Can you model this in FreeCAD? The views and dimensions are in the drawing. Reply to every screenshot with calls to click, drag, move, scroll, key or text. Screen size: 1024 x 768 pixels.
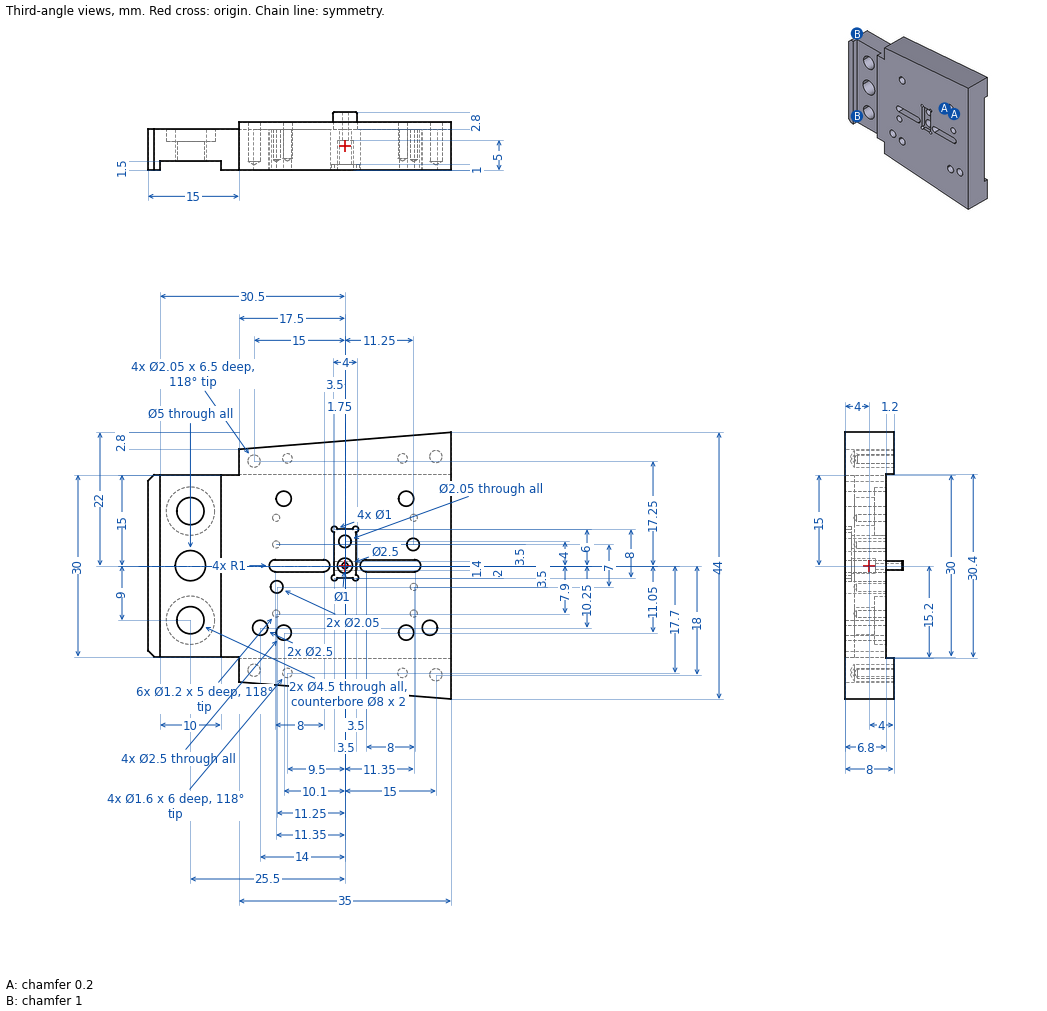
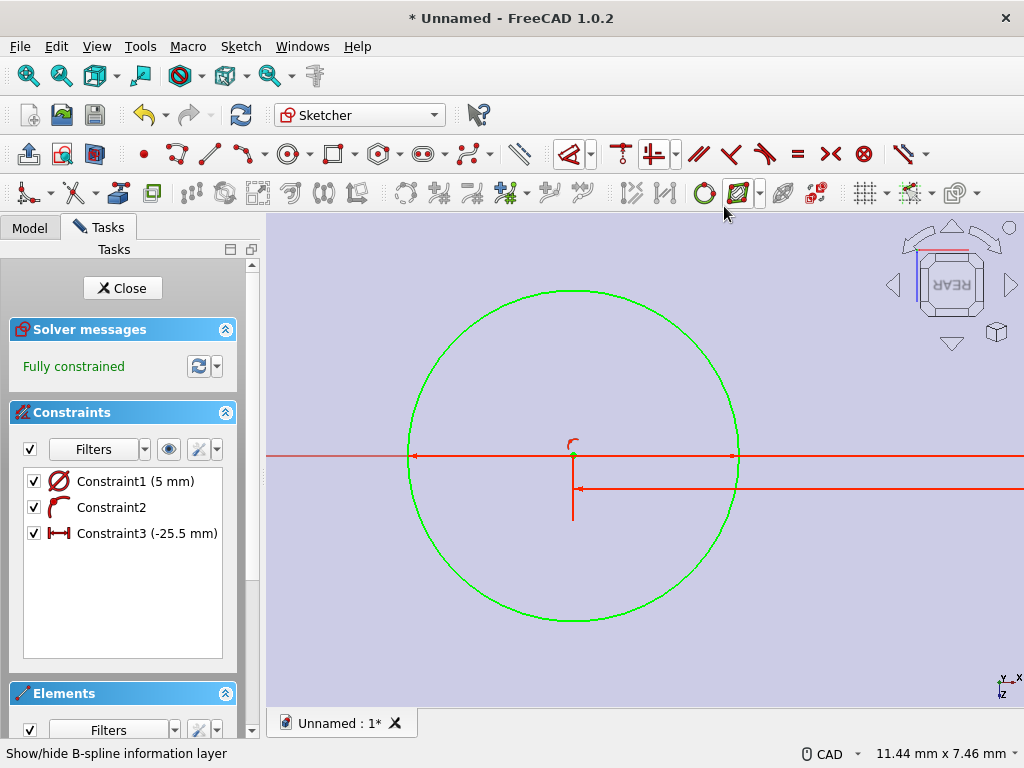
click(123, 288)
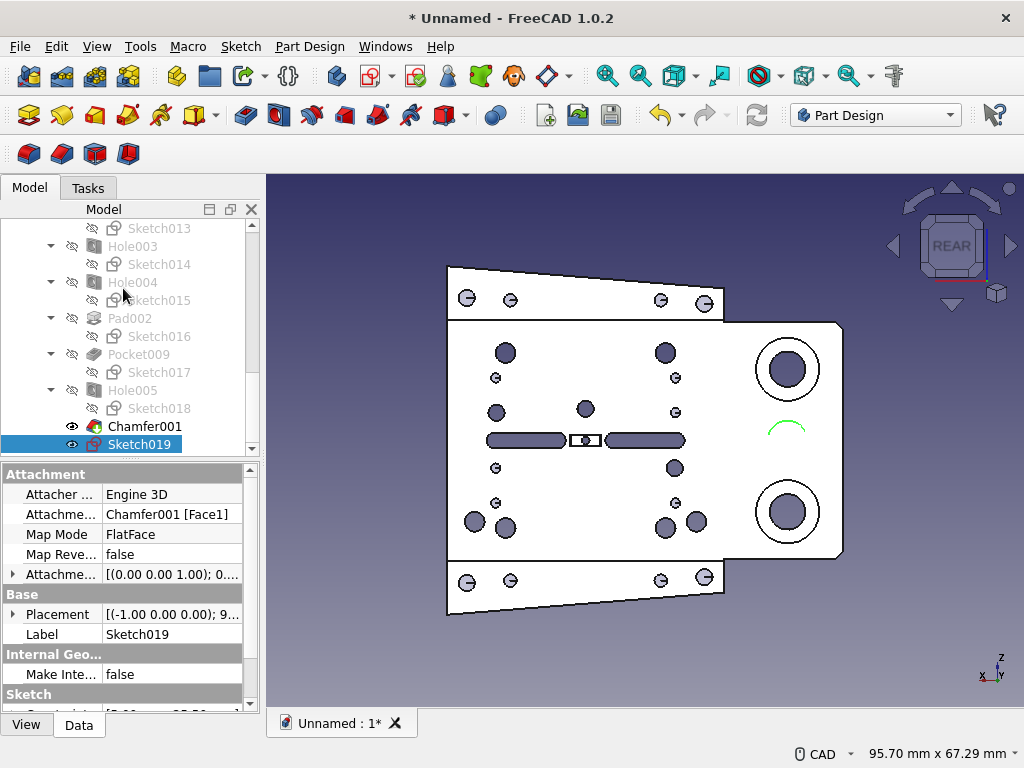
click(279, 116)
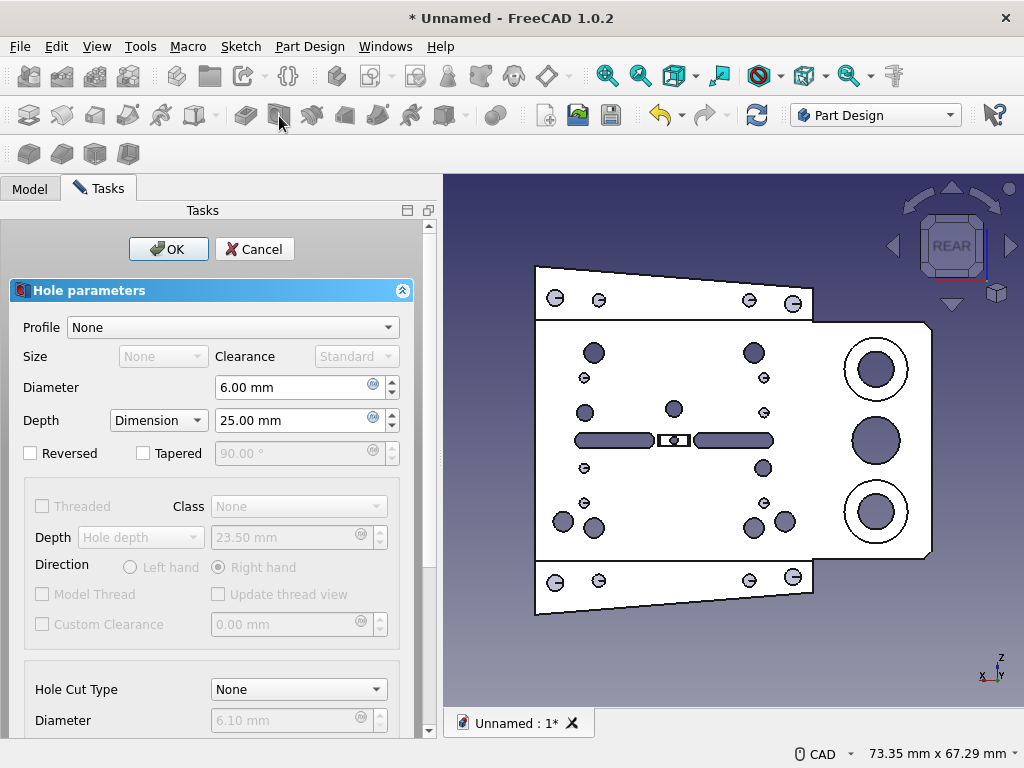
triple_click(300, 388)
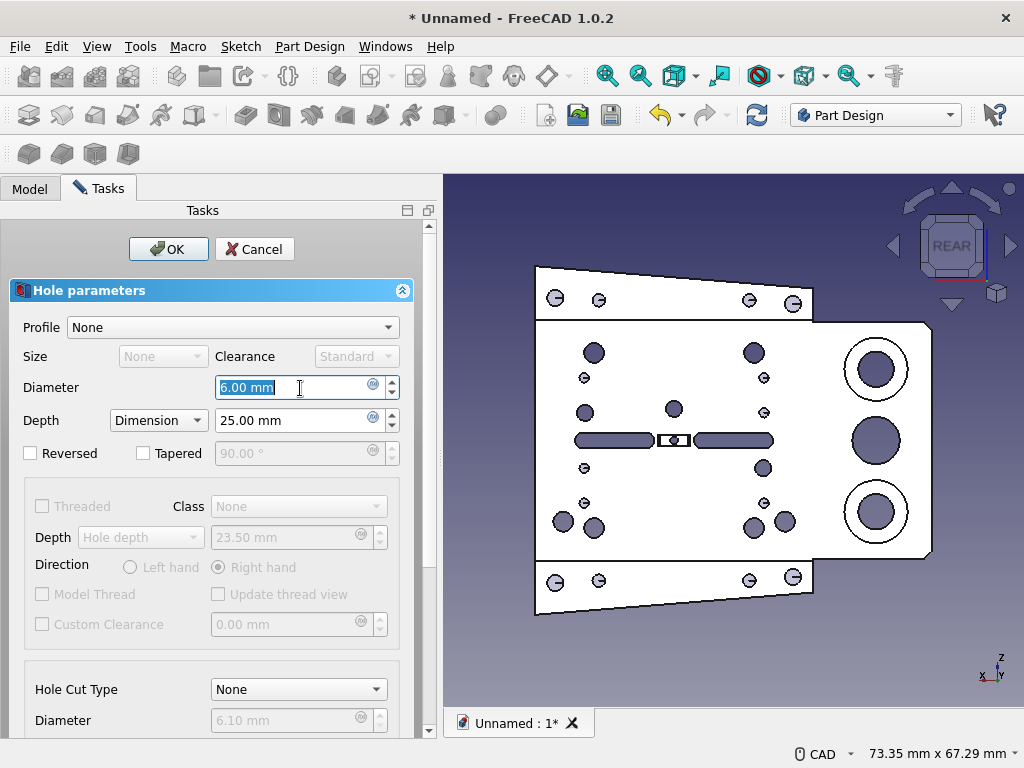
text(5)
key(Tab)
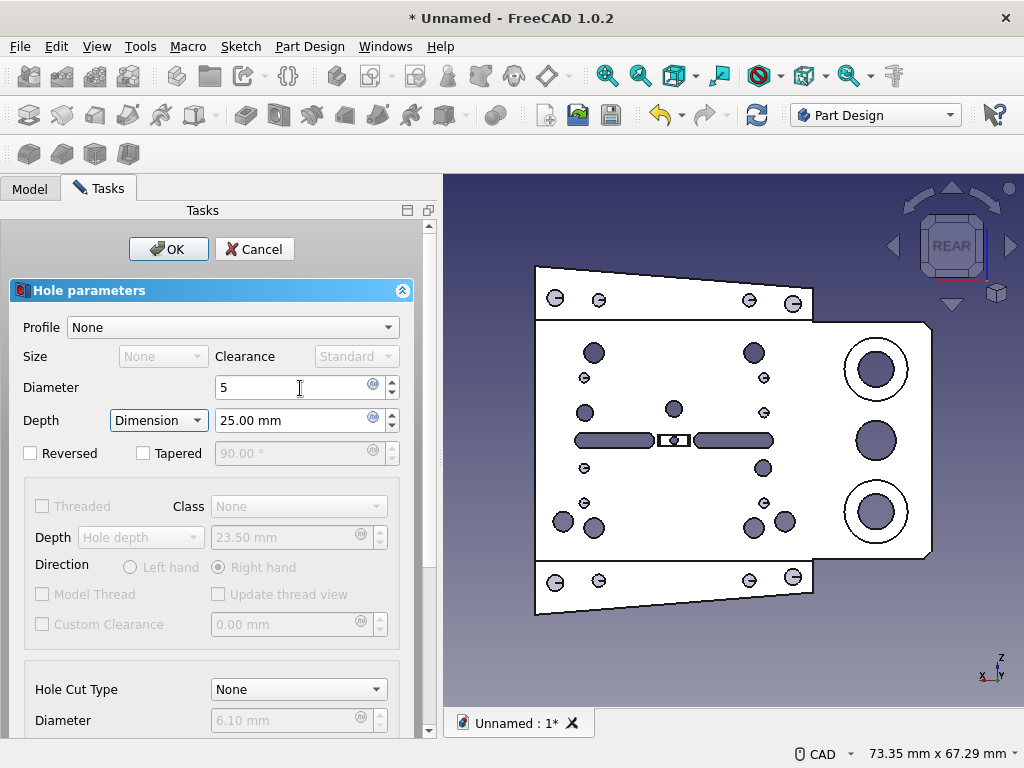
click(160, 420)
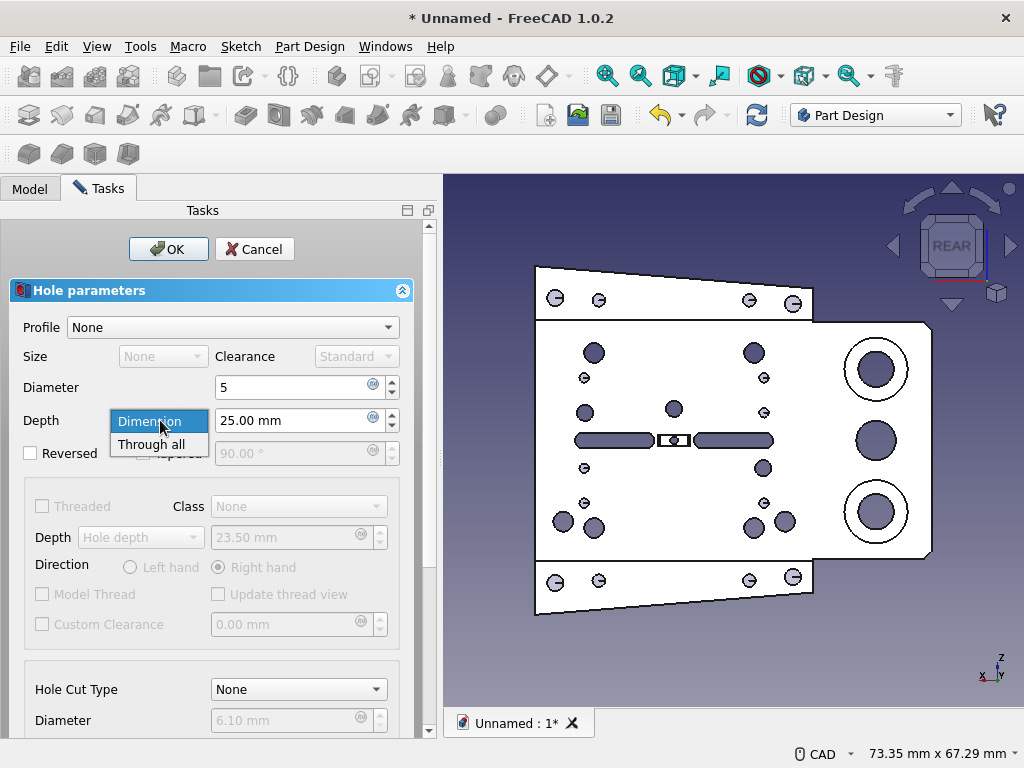
click(158, 444)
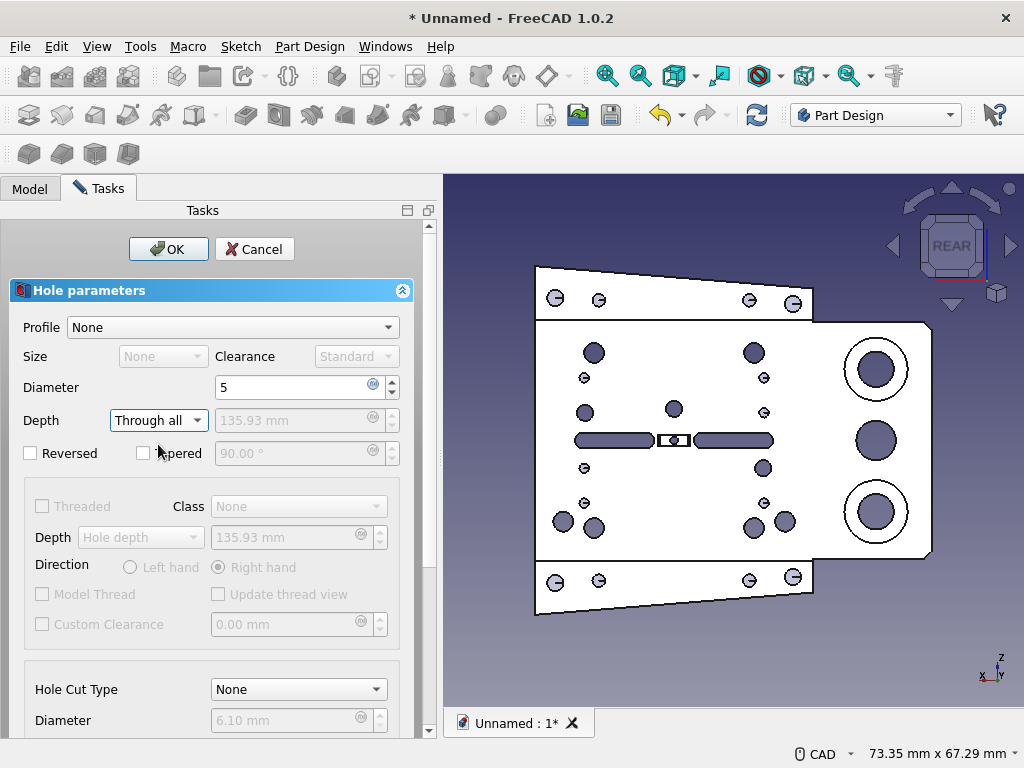
click(169, 249)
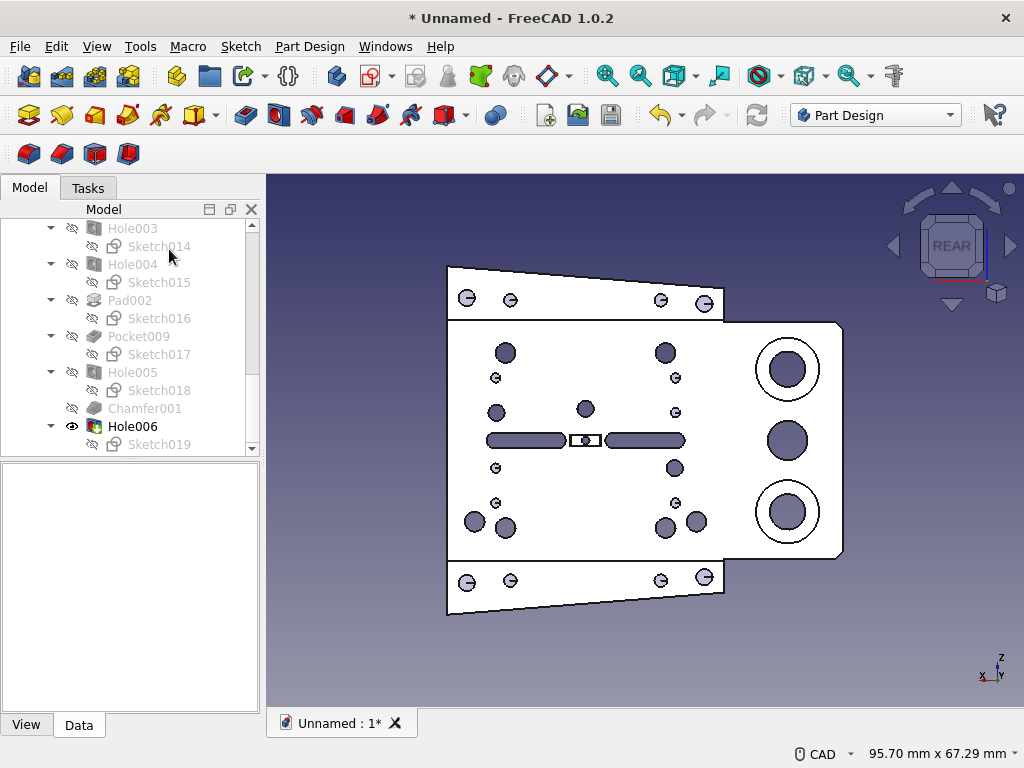
key(0)